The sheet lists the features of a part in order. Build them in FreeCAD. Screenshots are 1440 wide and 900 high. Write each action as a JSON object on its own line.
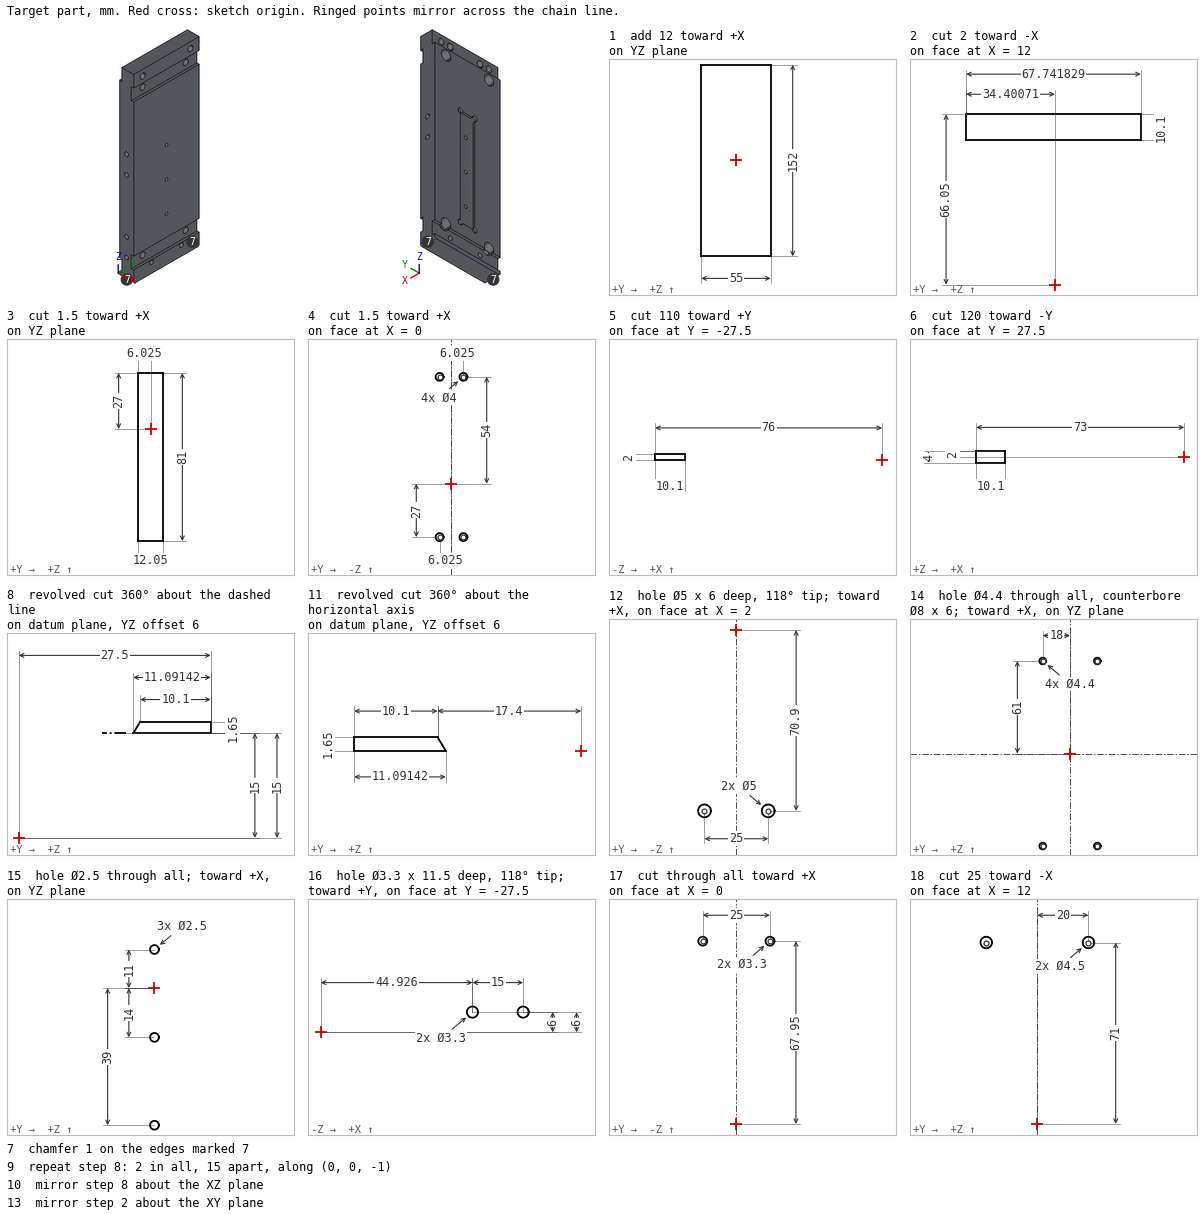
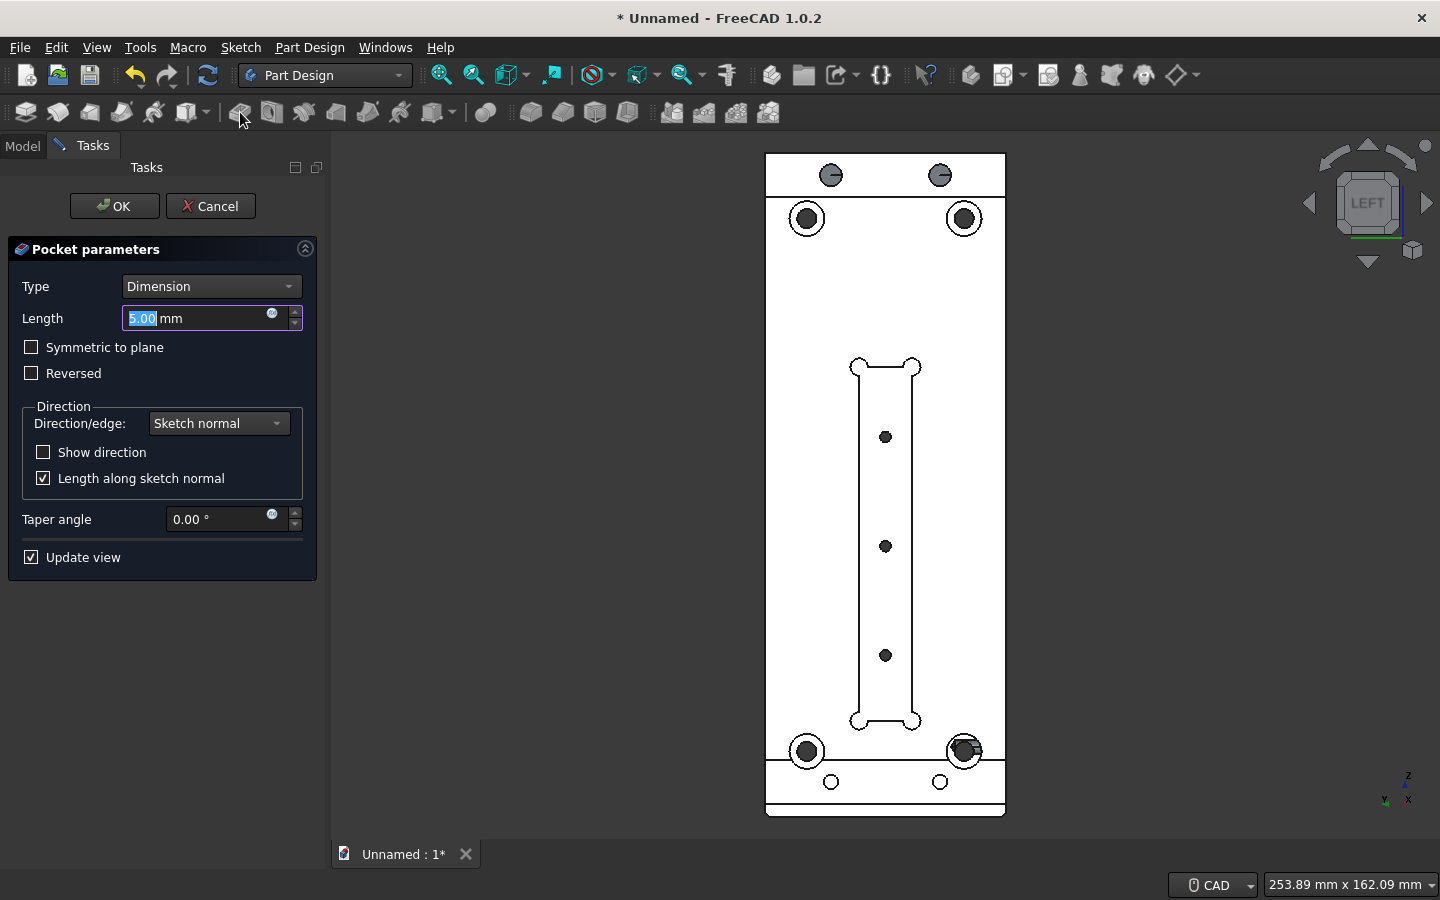
{"action": "left_click", "coordinate": [212, 286]}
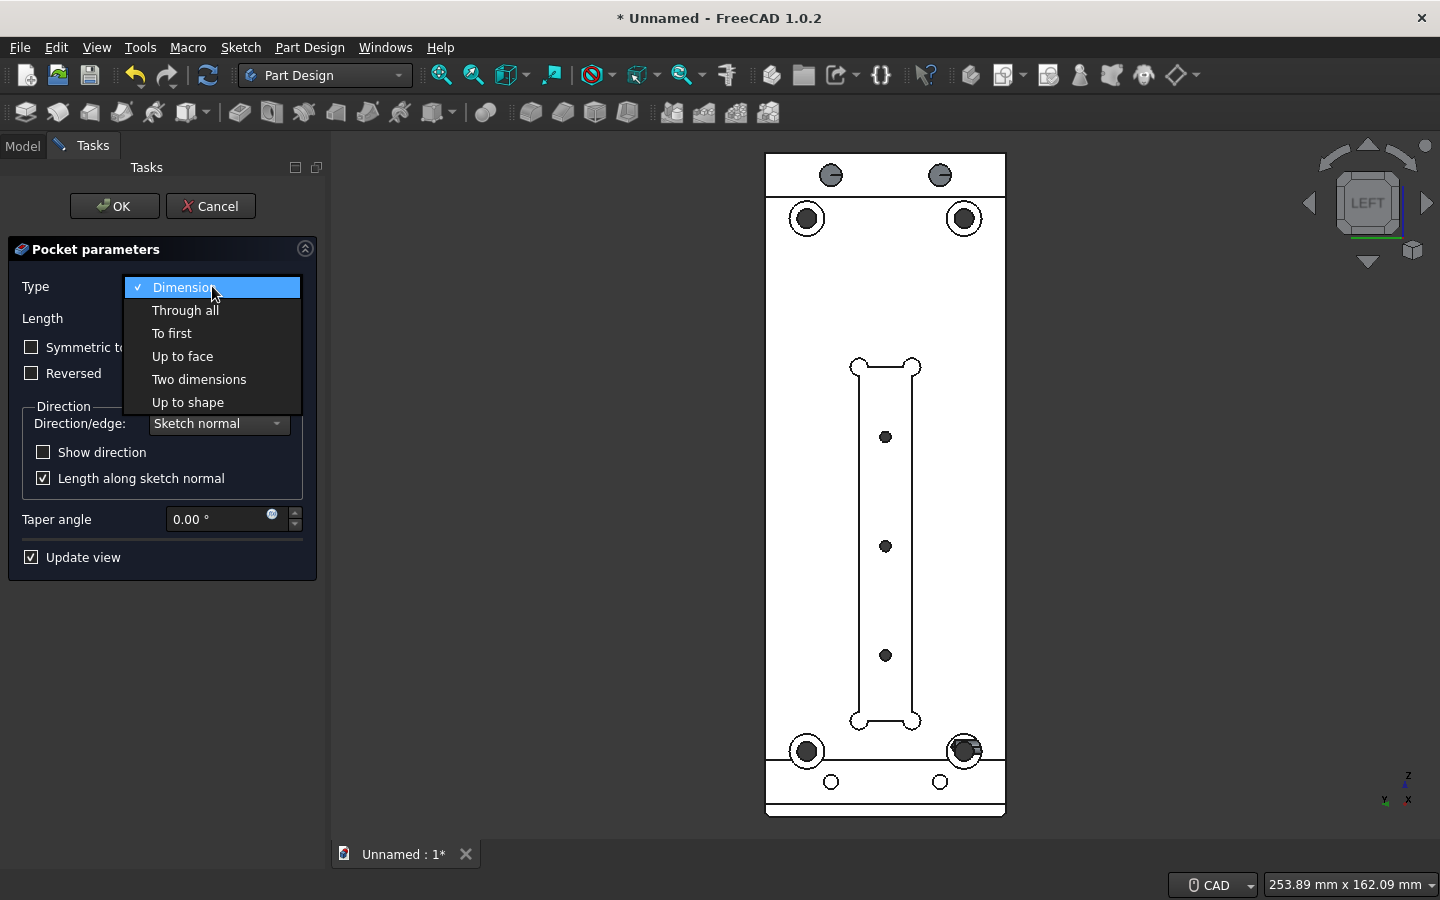
{"action": "left_click", "coordinate": [212, 310]}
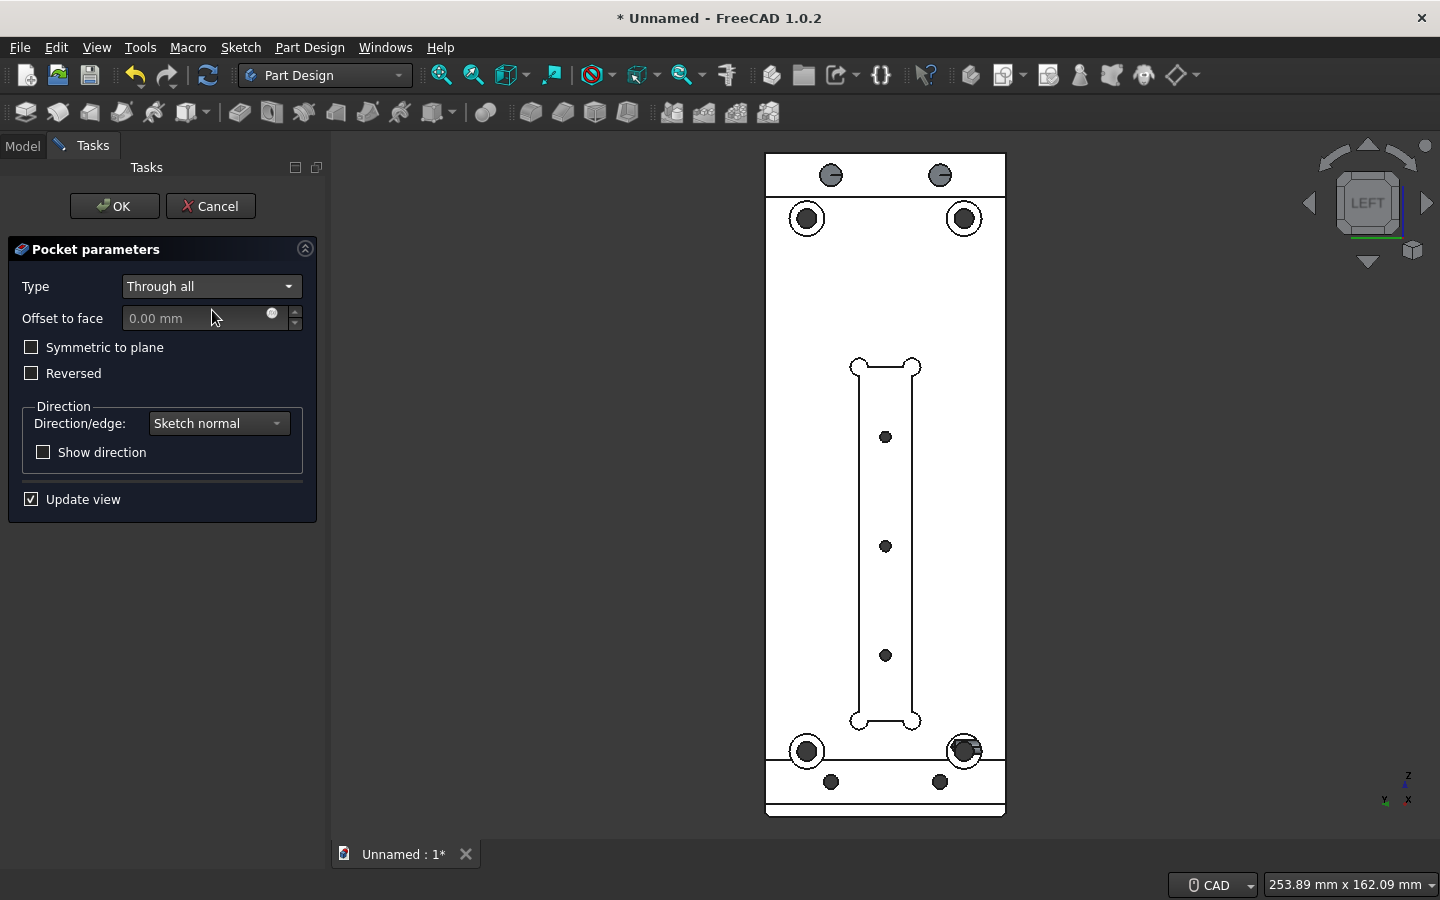
{"action": "left_click", "coordinate": [115, 206]}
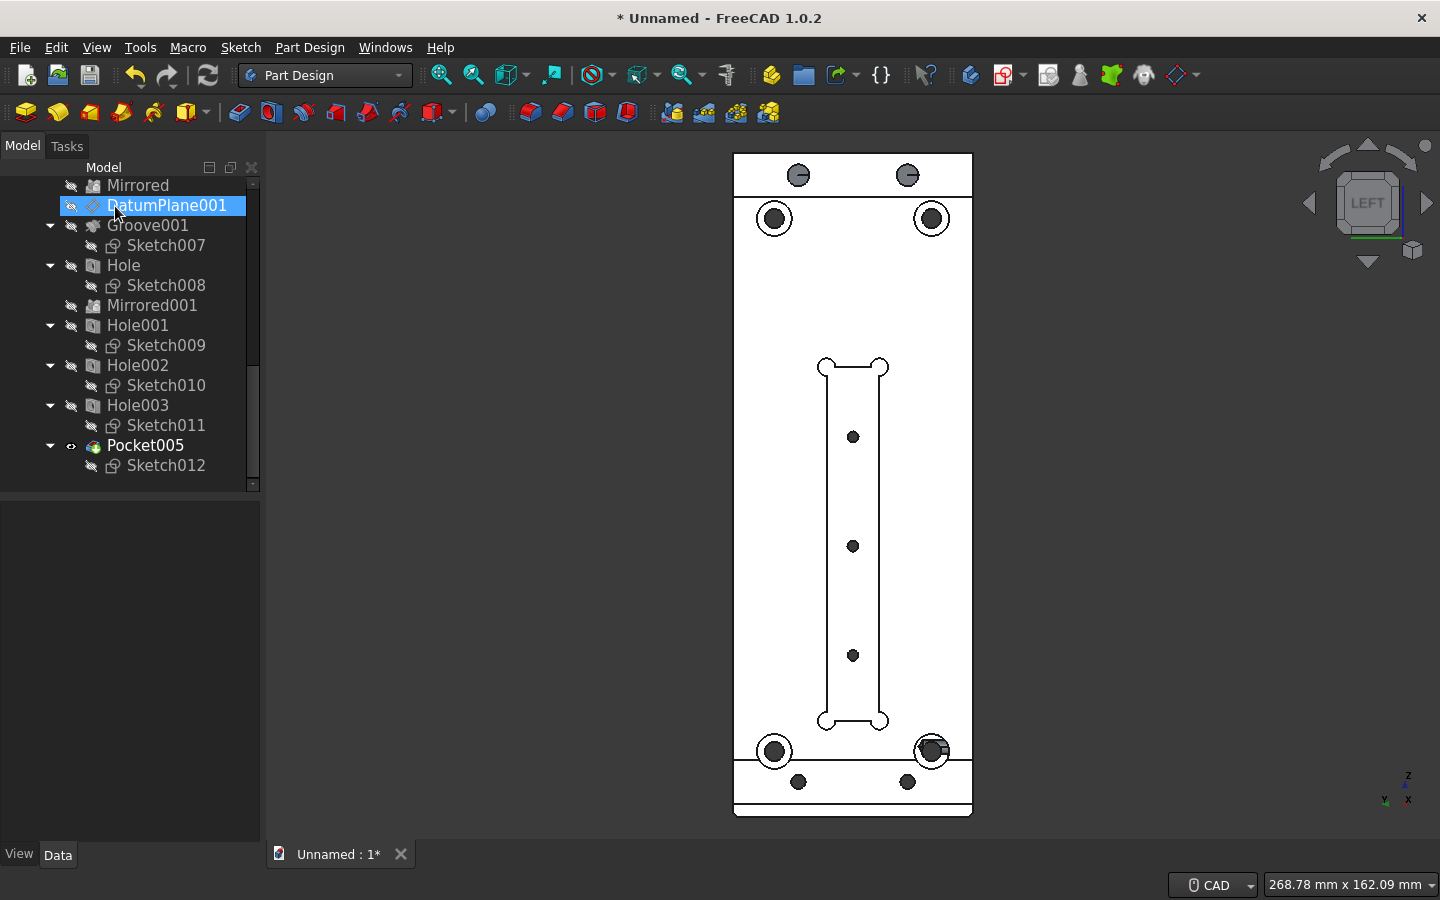
{"action": "key", "text": "0"}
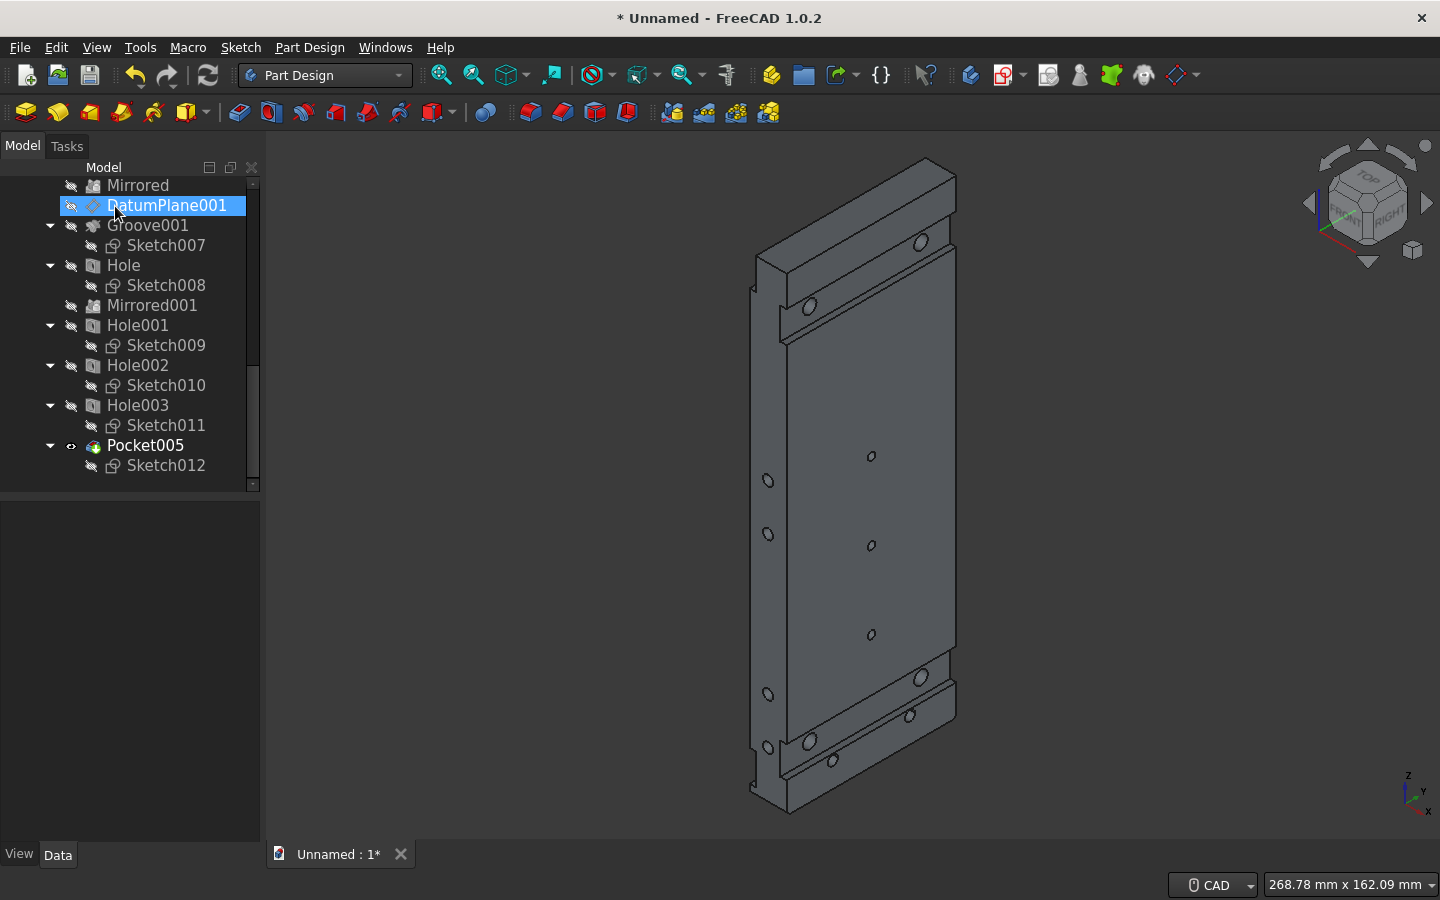
{"action": "left_click", "coordinate": [872, 381]}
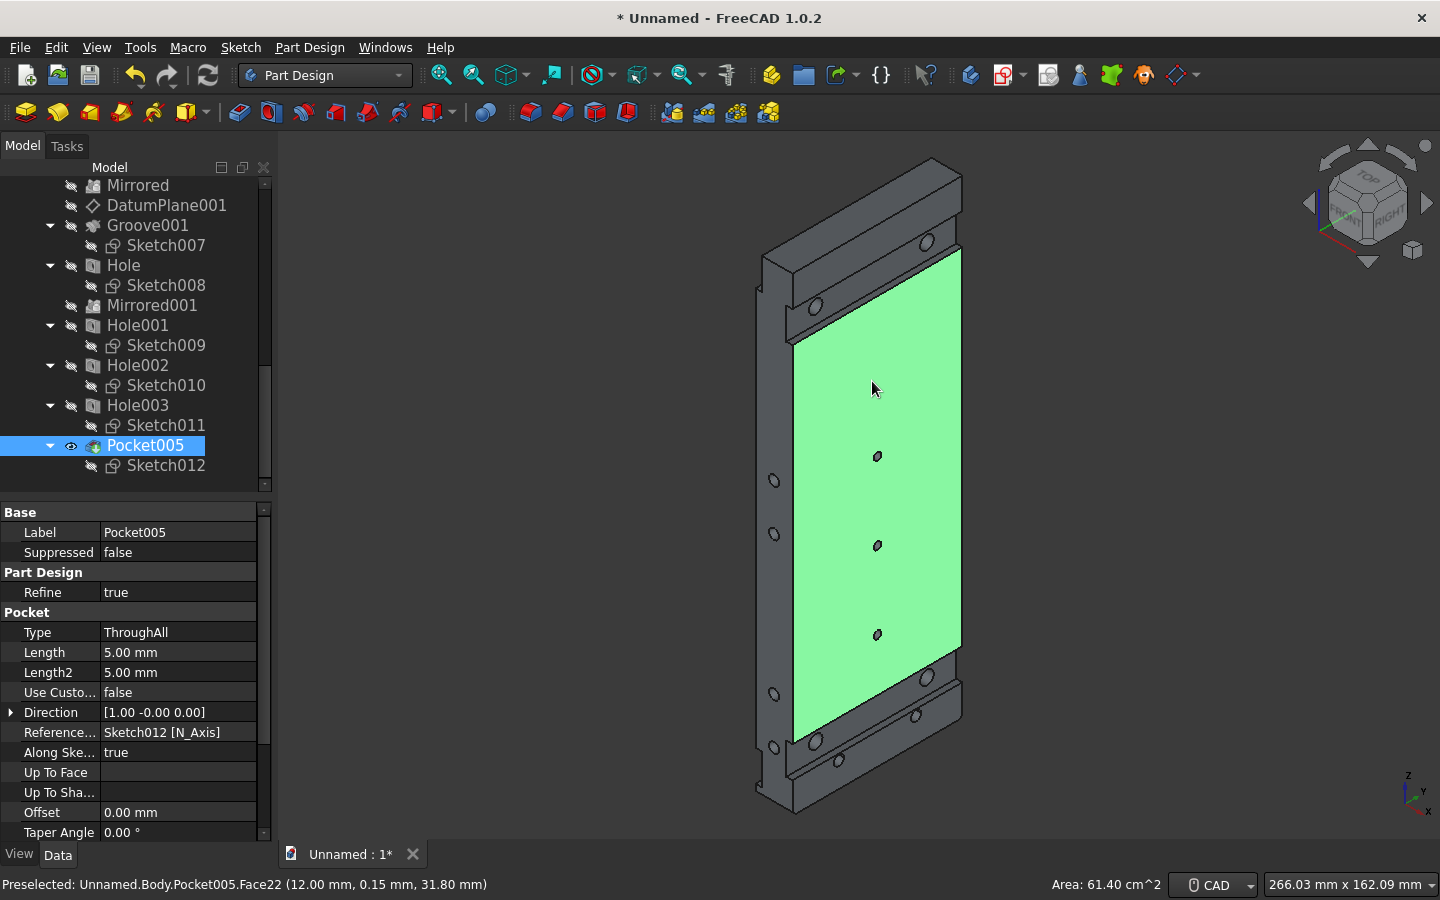
{"action": "left_click", "coordinate": [1004, 76]}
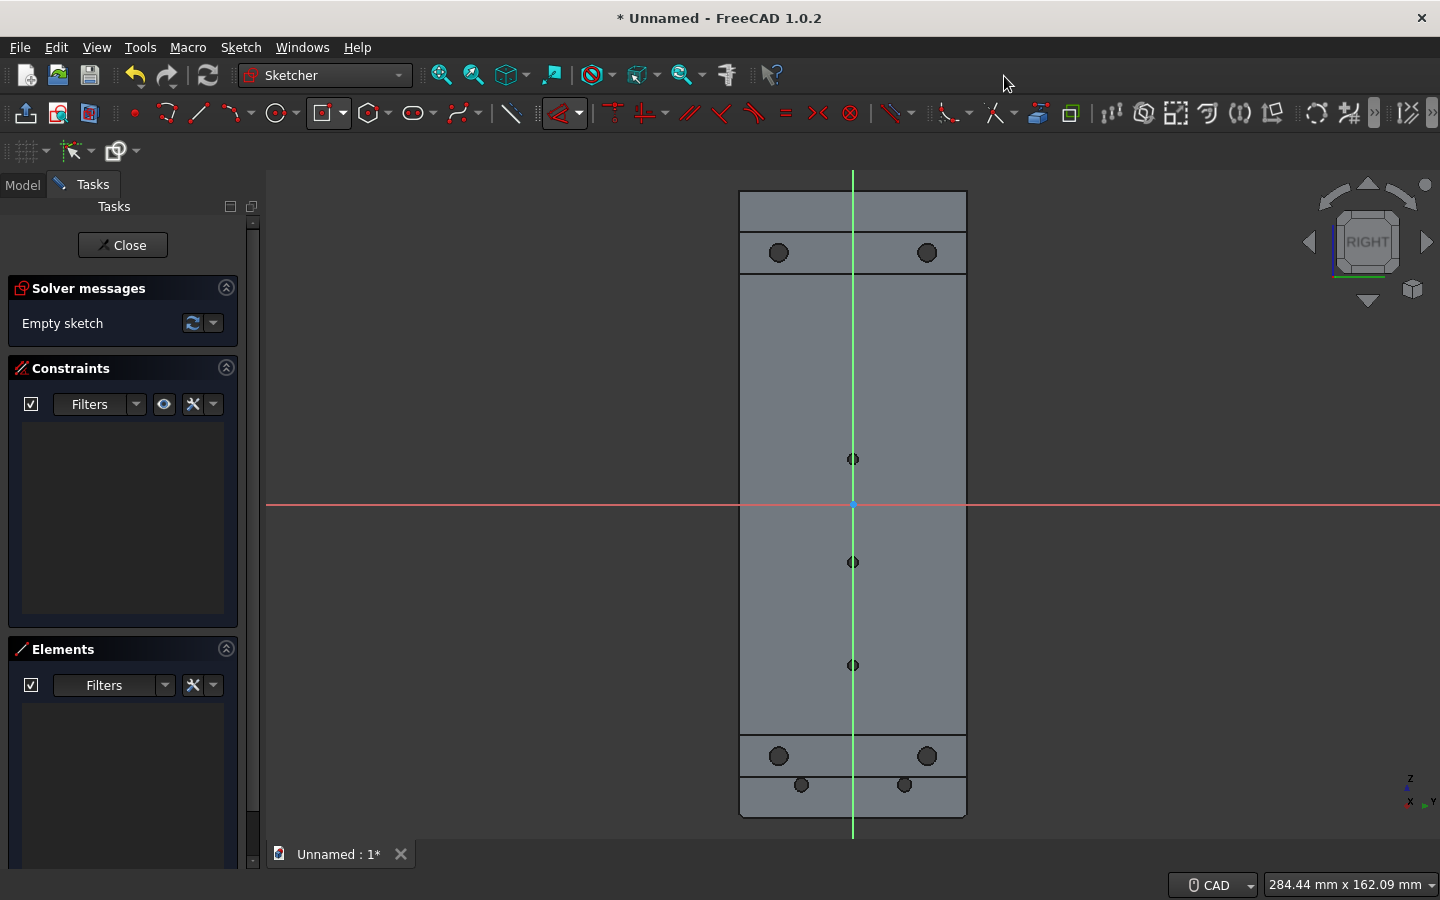
{"action": "scroll", "coordinate": [475, 811], "scroll_direction": "down", "scroll_amount": 1}